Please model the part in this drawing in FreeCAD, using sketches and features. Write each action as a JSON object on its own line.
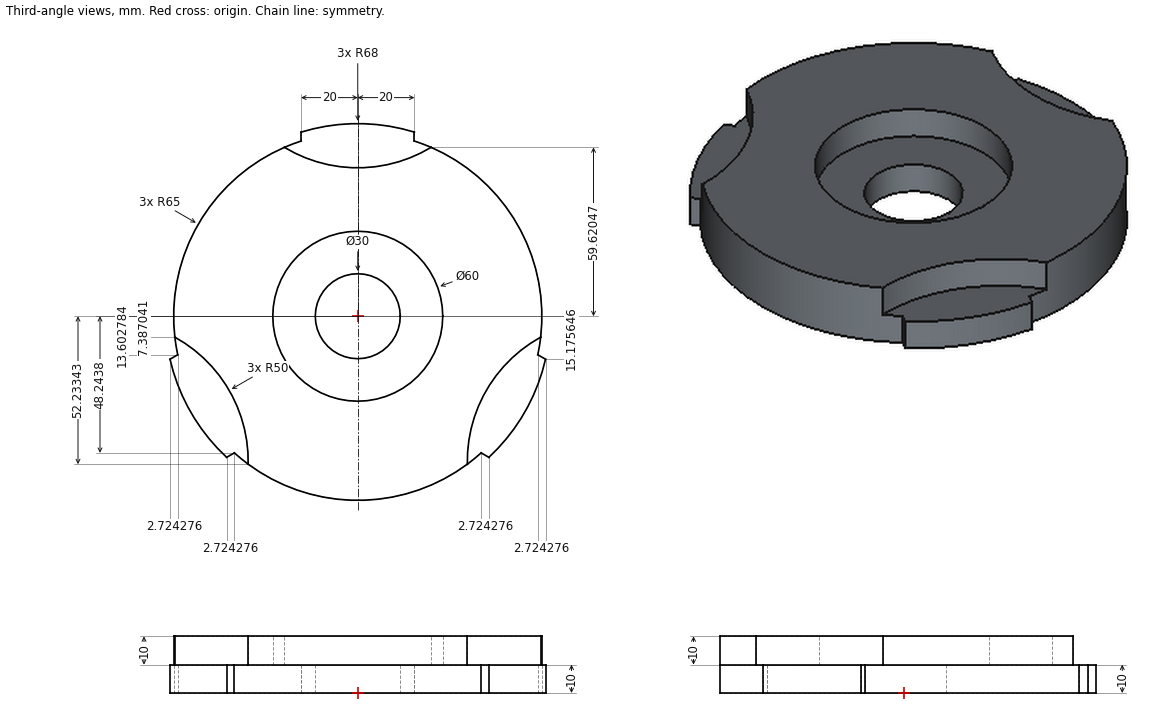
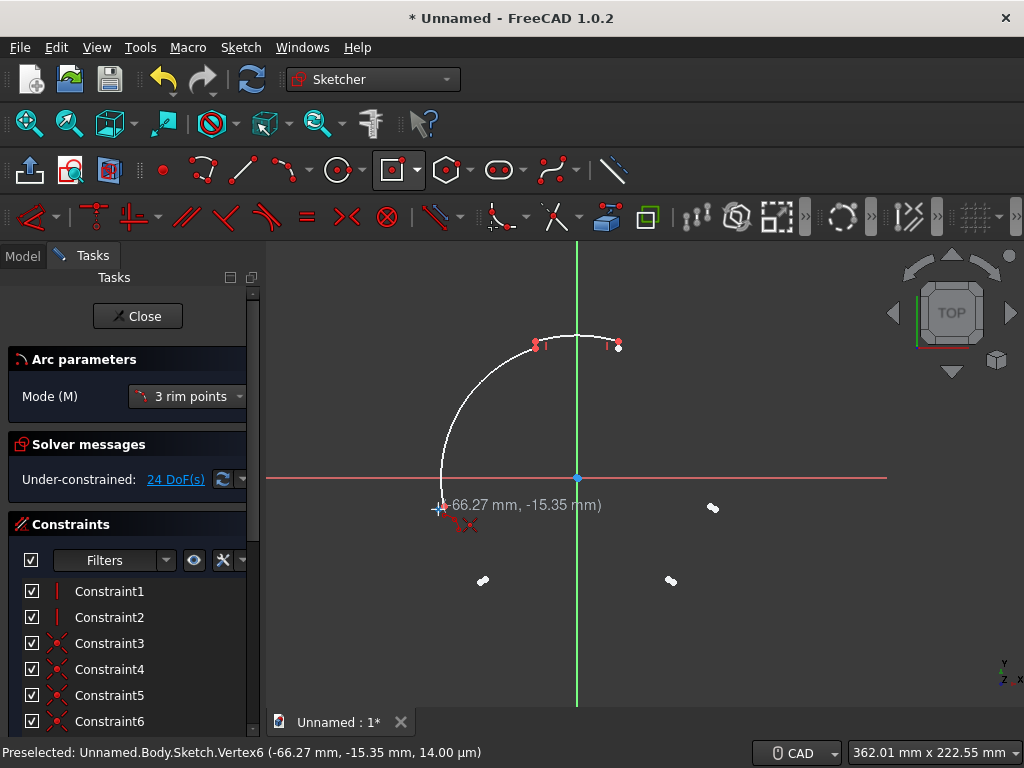
{"action": "scroll", "coordinate": [480, 582], "scroll_direction": "up", "scroll_amount": 8}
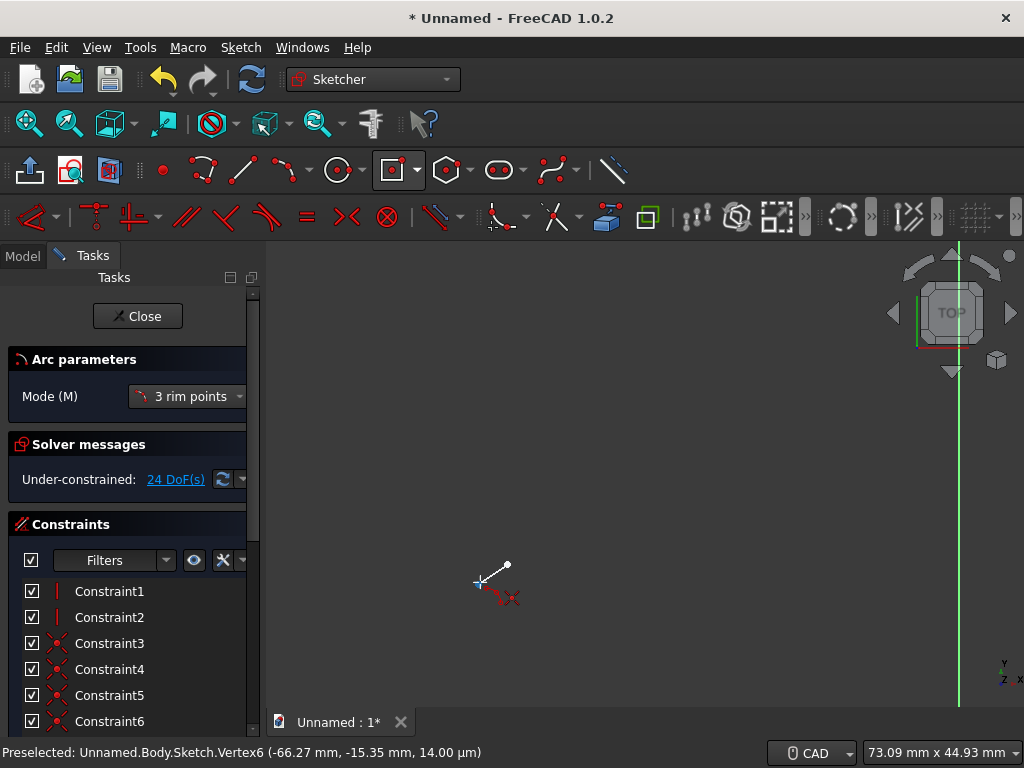
{"action": "left_click", "coordinate": [479, 584]}
{"action": "left_click", "coordinate": [348, 415]}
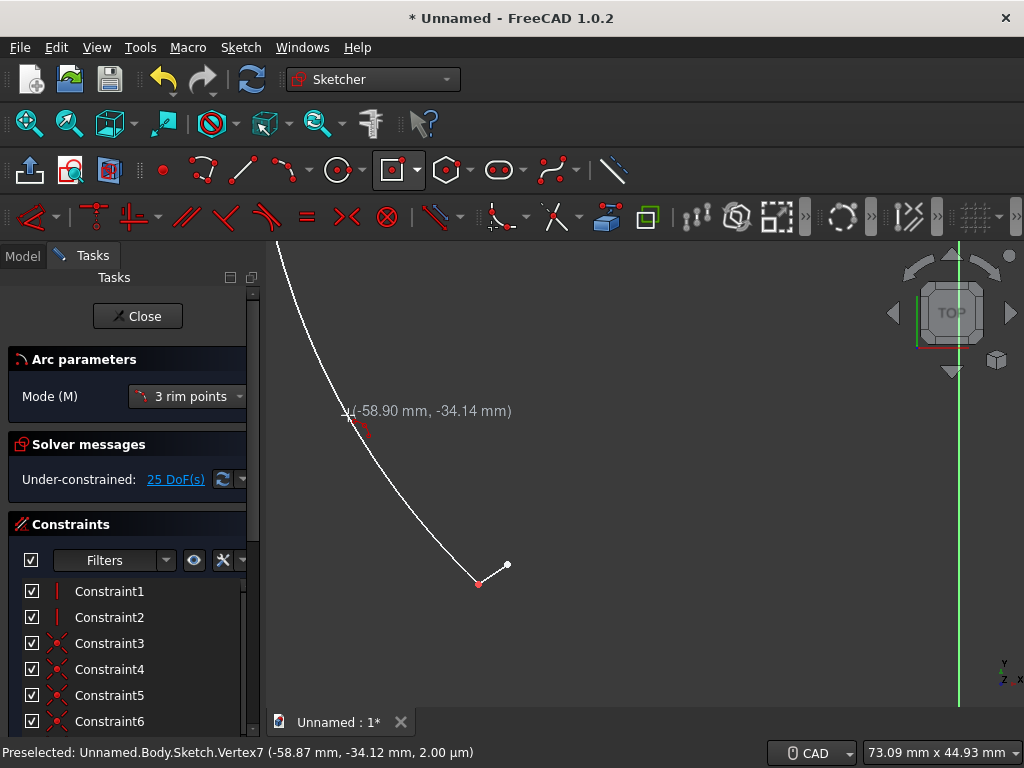
{"action": "left_click", "coordinate": [508, 565]}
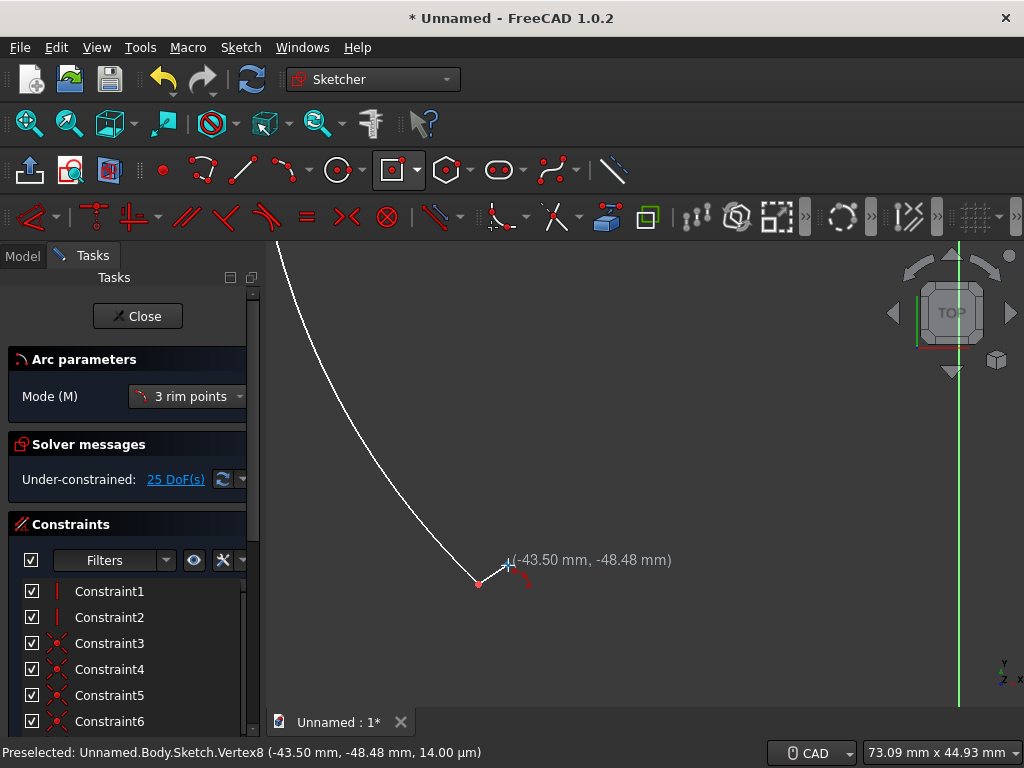
{"action": "scroll", "coordinate": [480, 582], "scroll_direction": "down", "scroll_amount": 8}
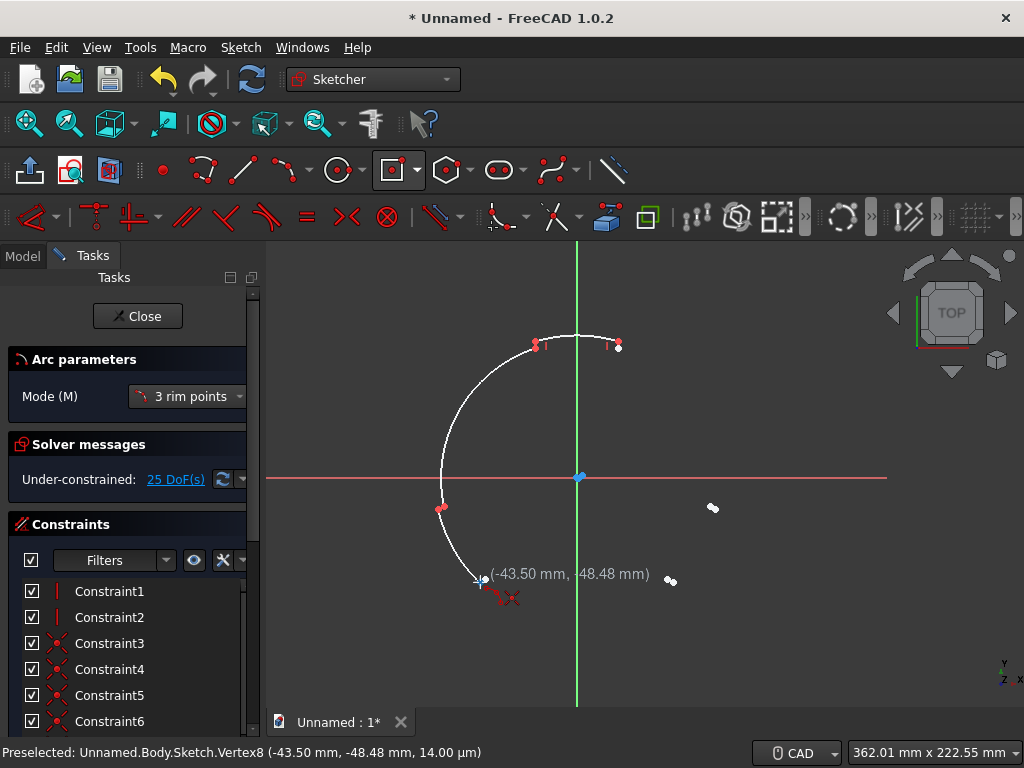
{"action": "scroll", "coordinate": [668, 579], "scroll_direction": "up", "scroll_amount": 8}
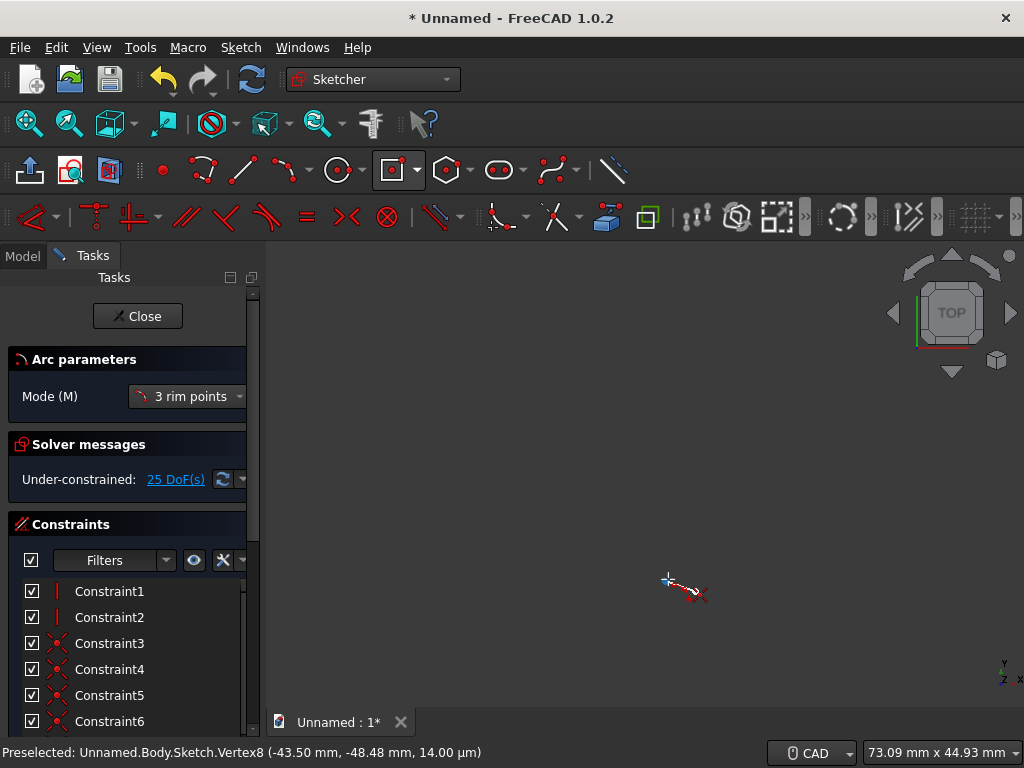
{"action": "left_click", "coordinate": [666, 581]}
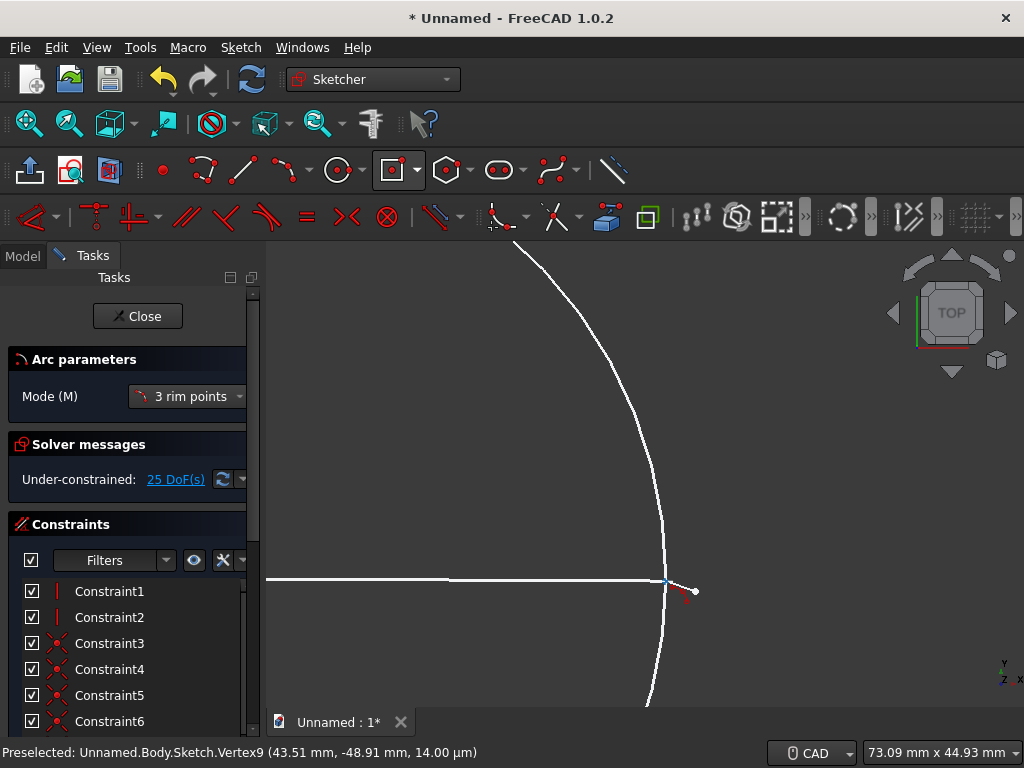
{"action": "scroll", "coordinate": [668, 579], "scroll_direction": "down", "scroll_amount": 8}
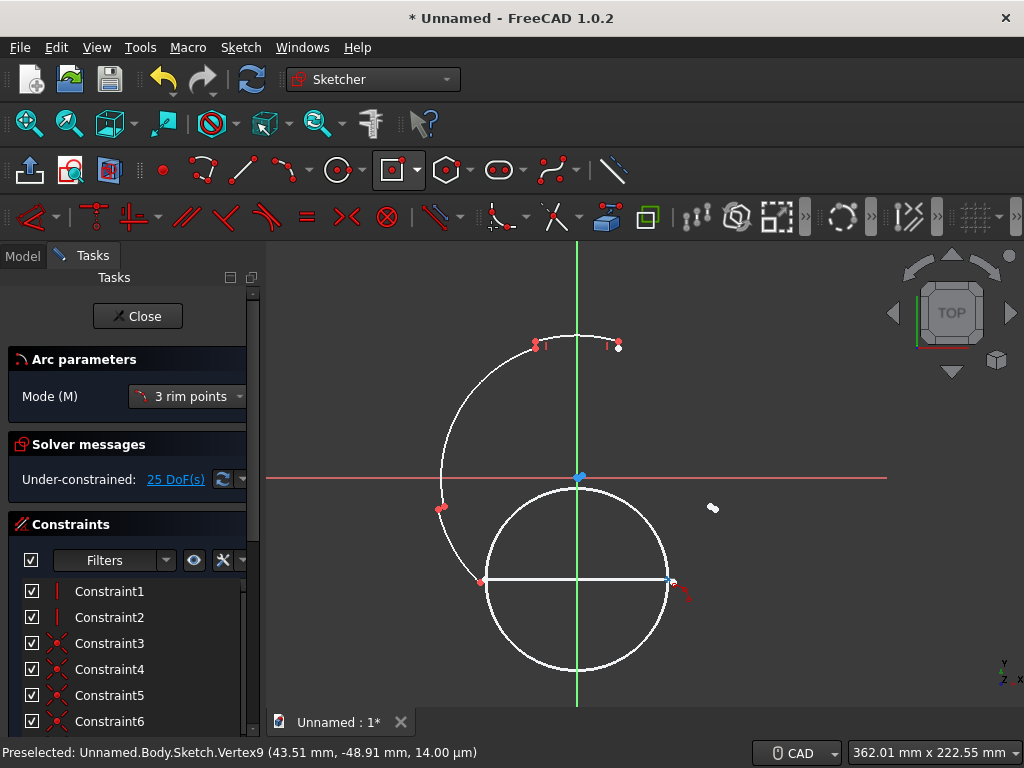
{"action": "left_click", "coordinate": [557, 612]}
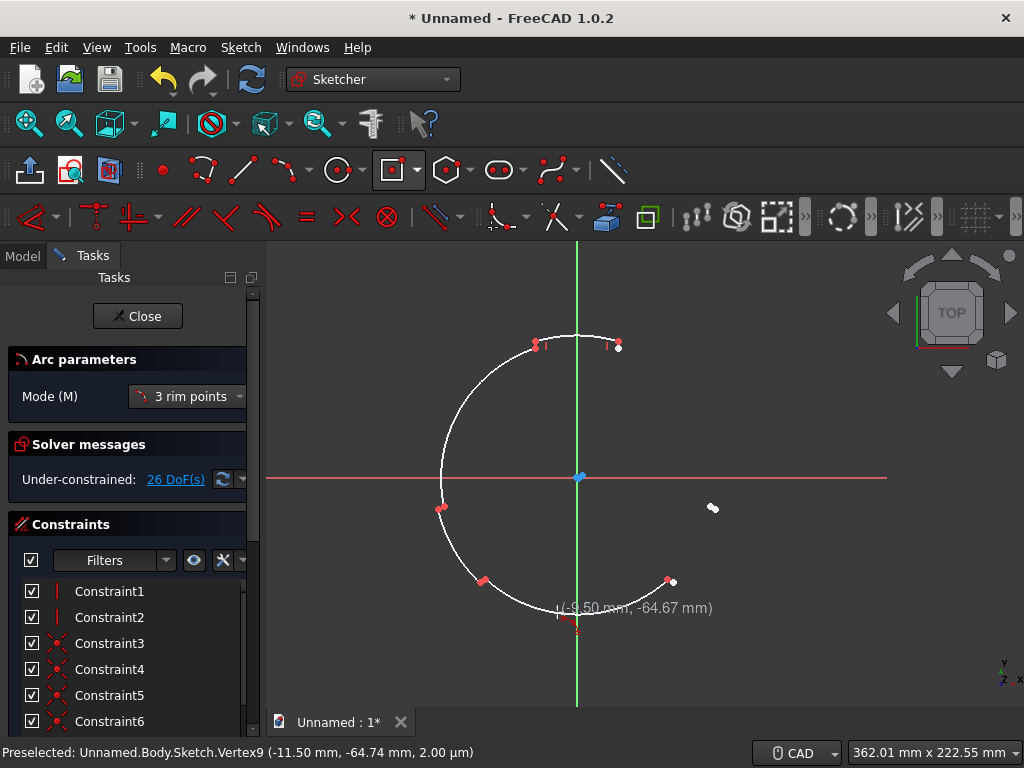
{"action": "scroll", "coordinate": [674, 582], "scroll_direction": "up", "scroll_amount": 8}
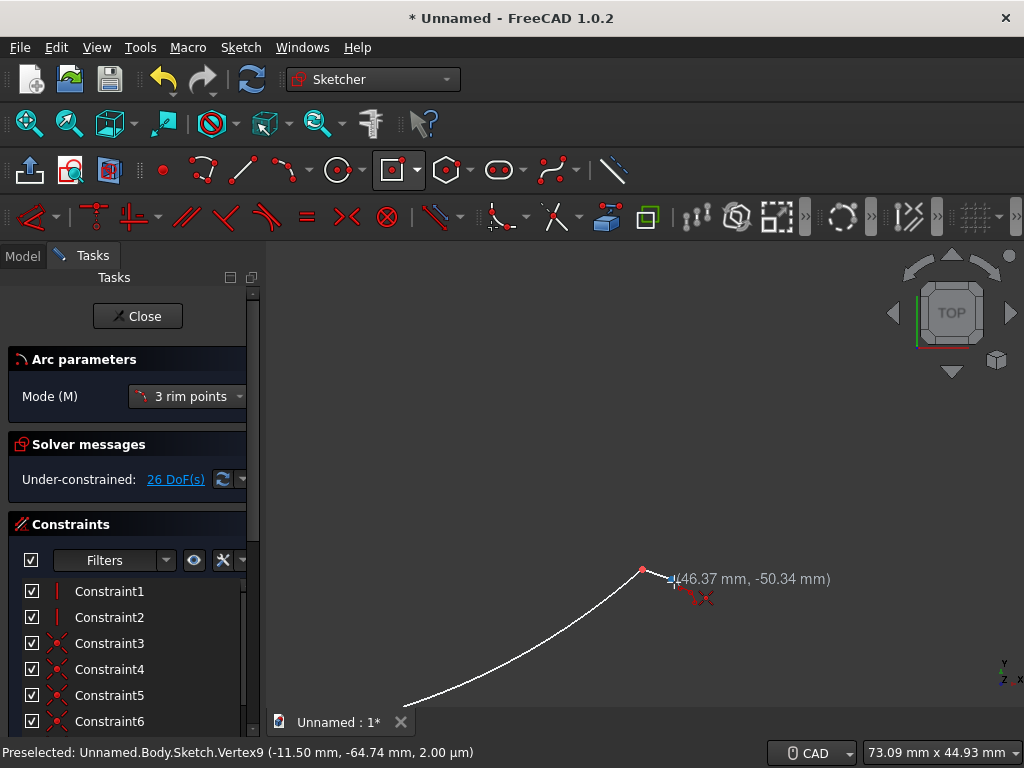
{"action": "left_click", "coordinate": [672, 580]}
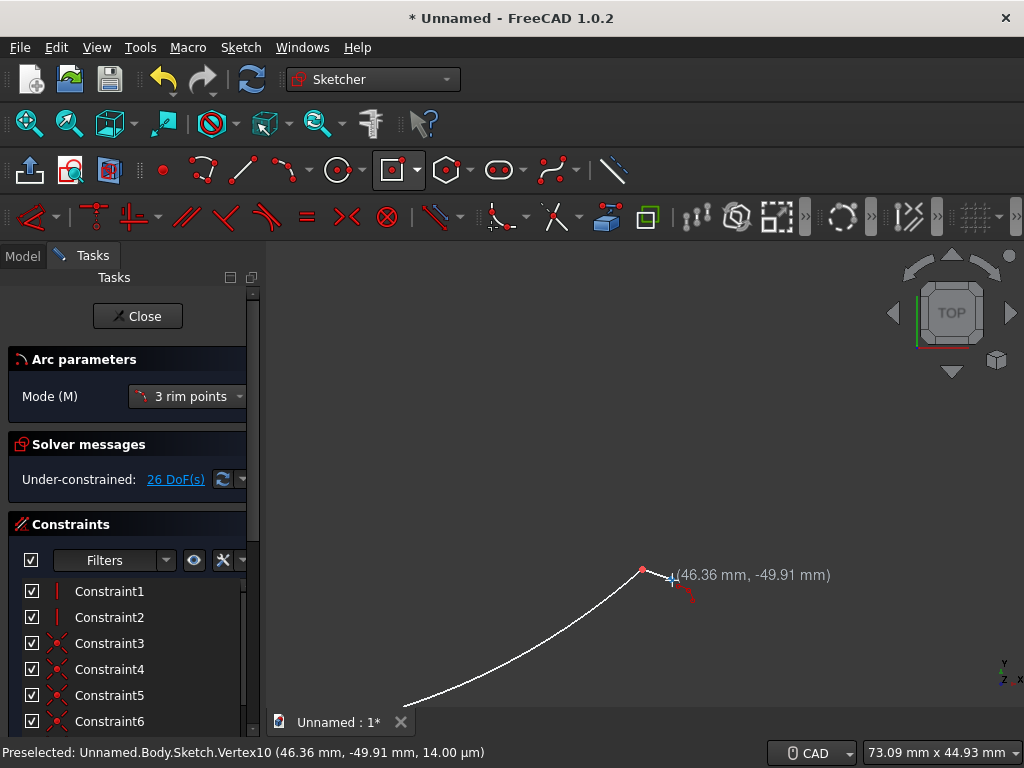
{"action": "scroll", "coordinate": [674, 582], "scroll_direction": "down", "scroll_amount": 8}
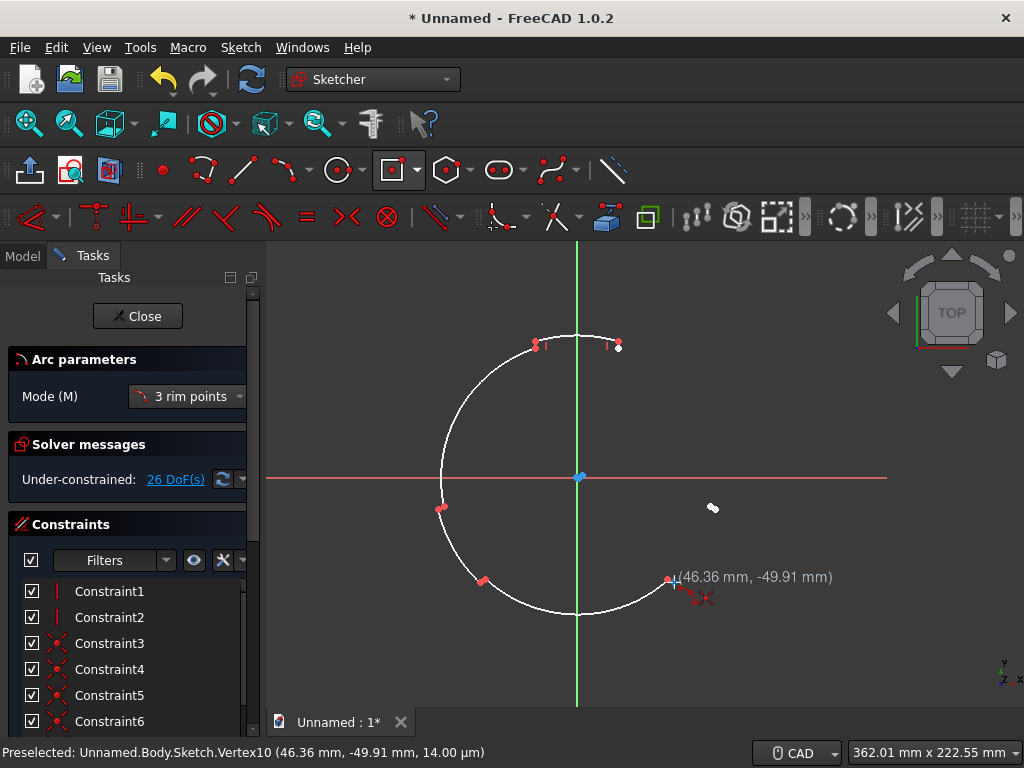
{"action": "scroll", "coordinate": [716, 509], "scroll_direction": "up", "scroll_amount": 8}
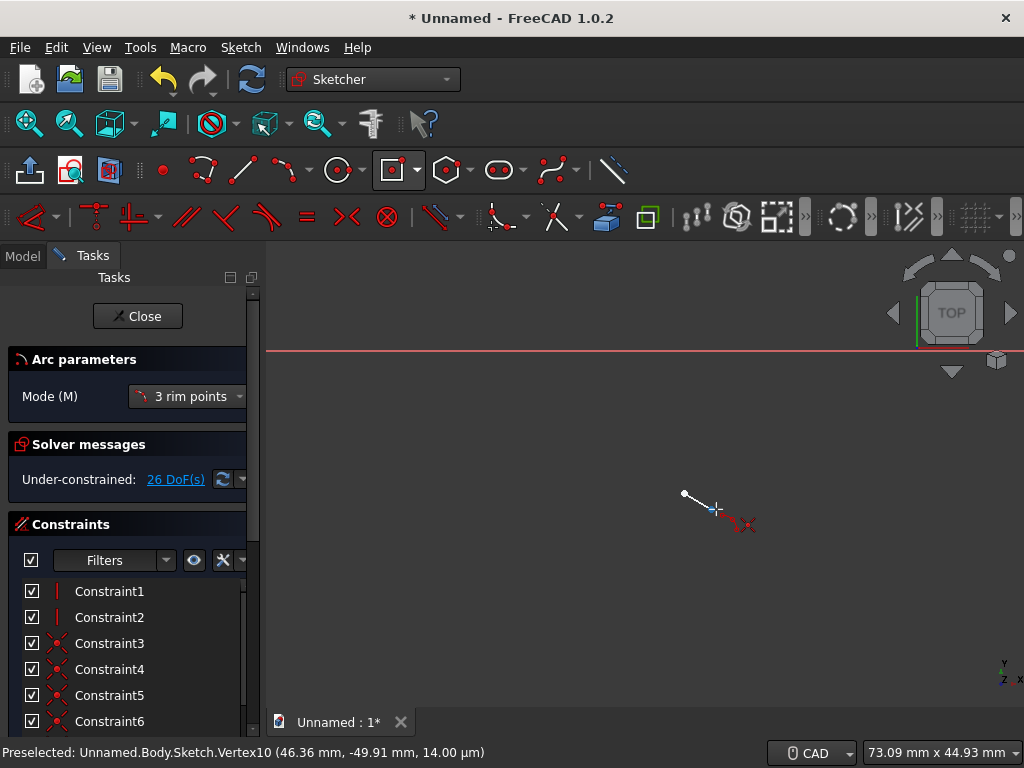
{"action": "left_click", "coordinate": [711, 510]}